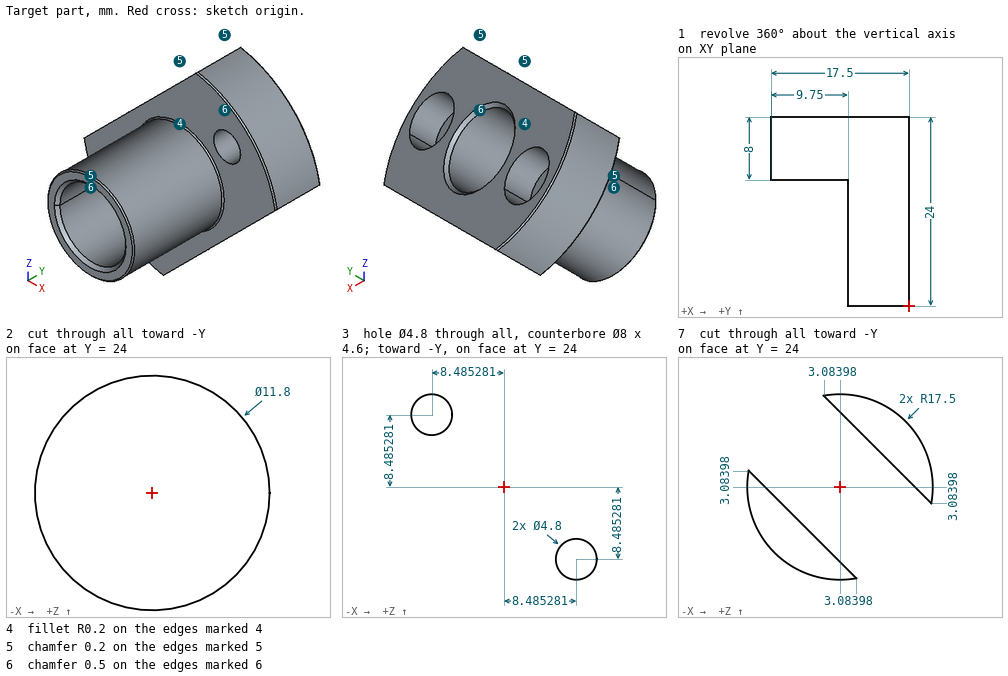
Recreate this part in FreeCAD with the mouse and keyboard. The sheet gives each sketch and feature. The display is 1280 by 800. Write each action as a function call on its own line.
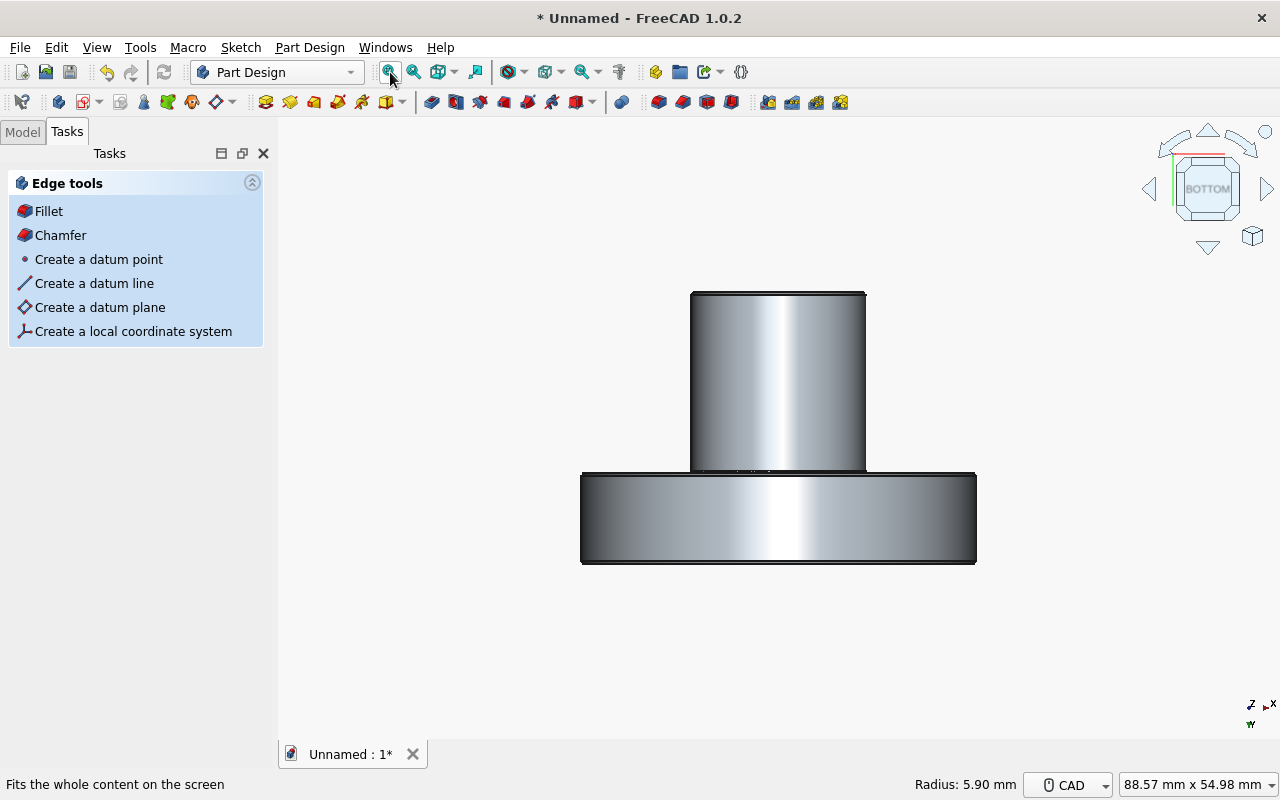
key(v)
key(f)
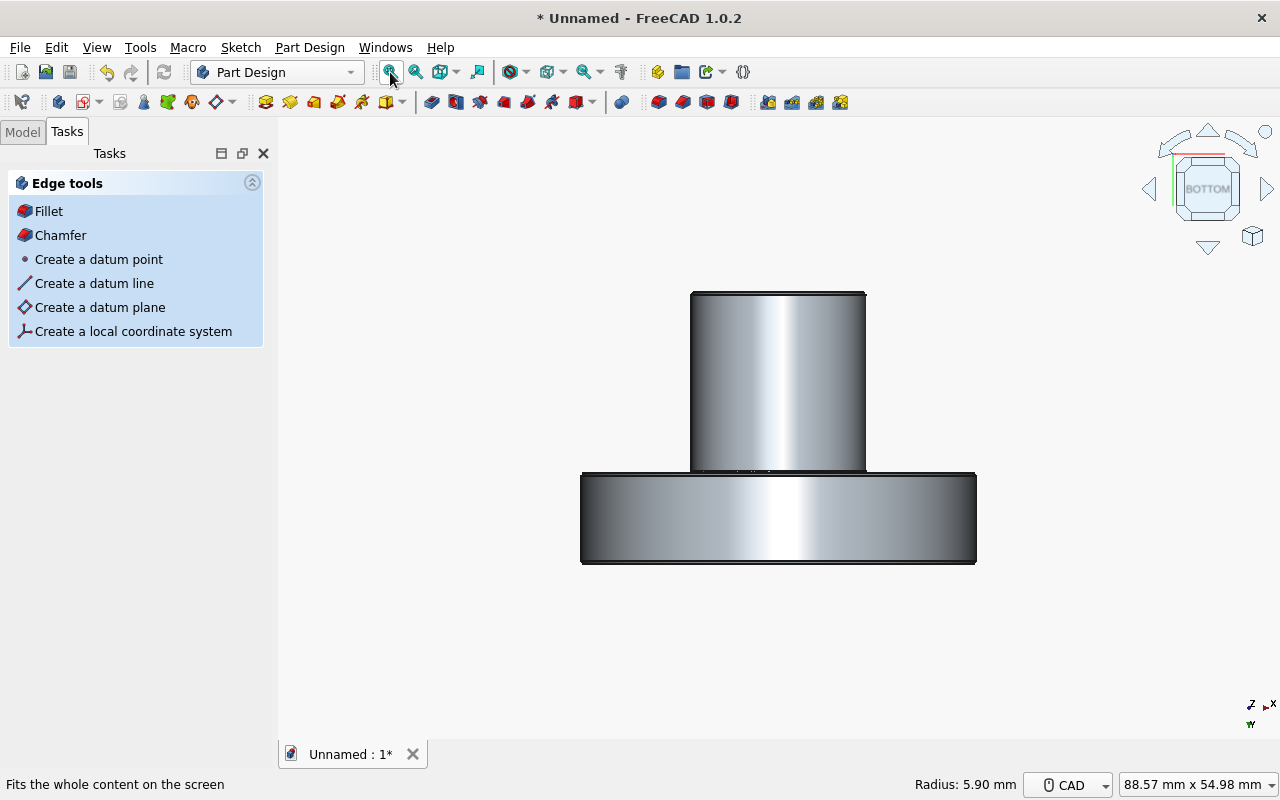
key(4)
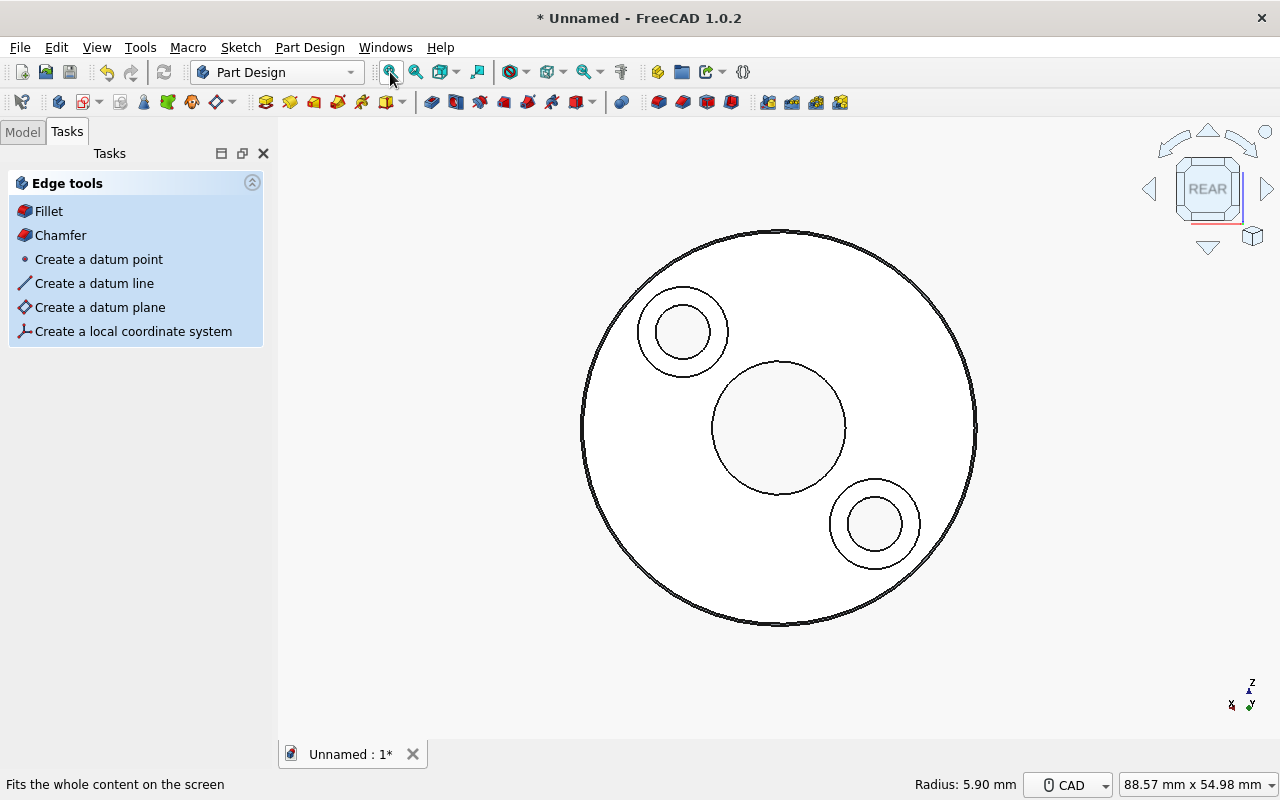
click(712, 427, ctrl)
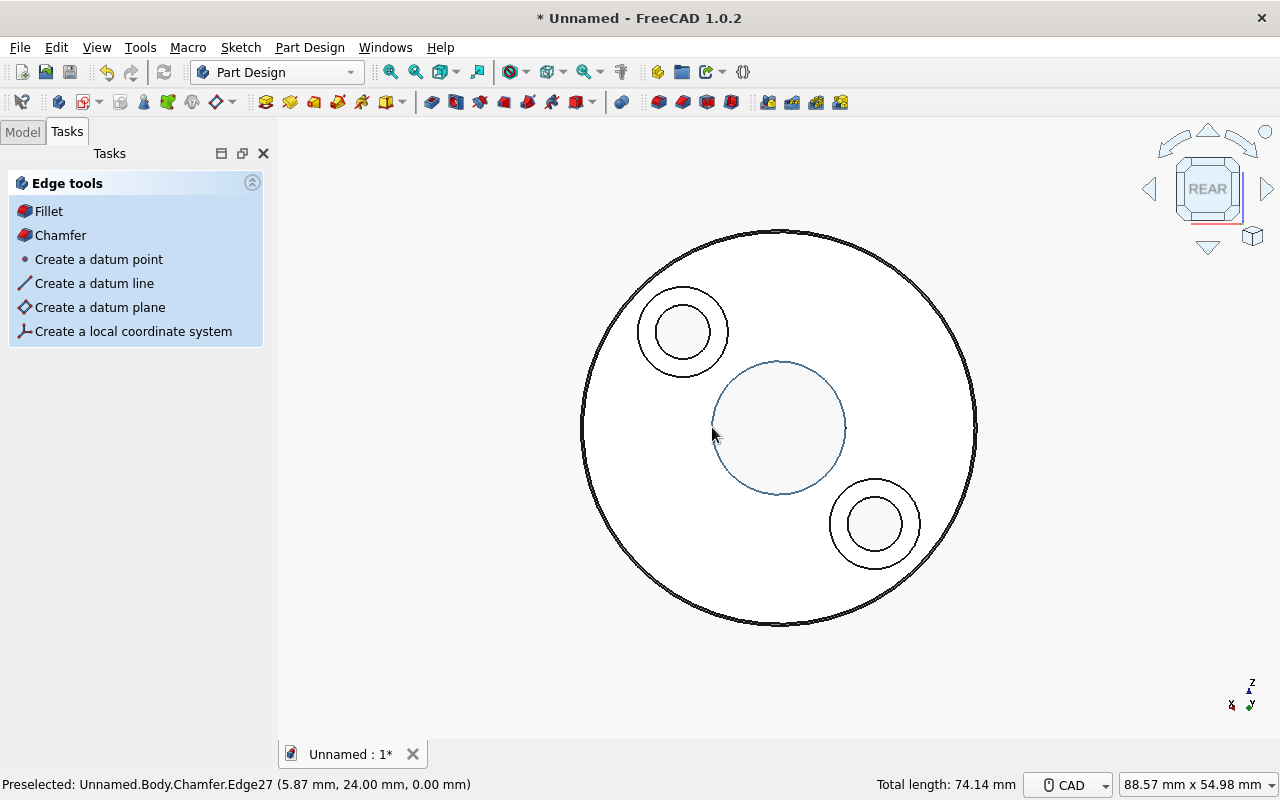
click(684, 102)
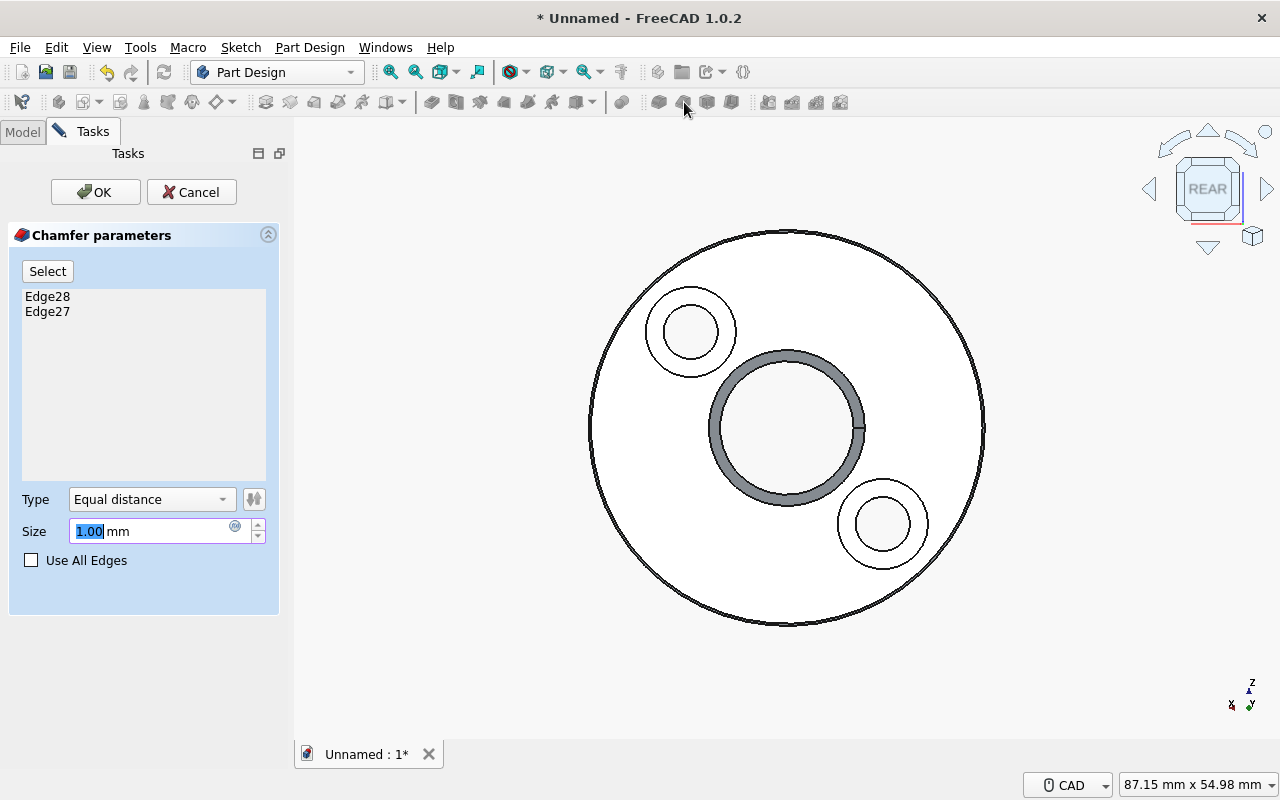
text(0.5)
key(Tab)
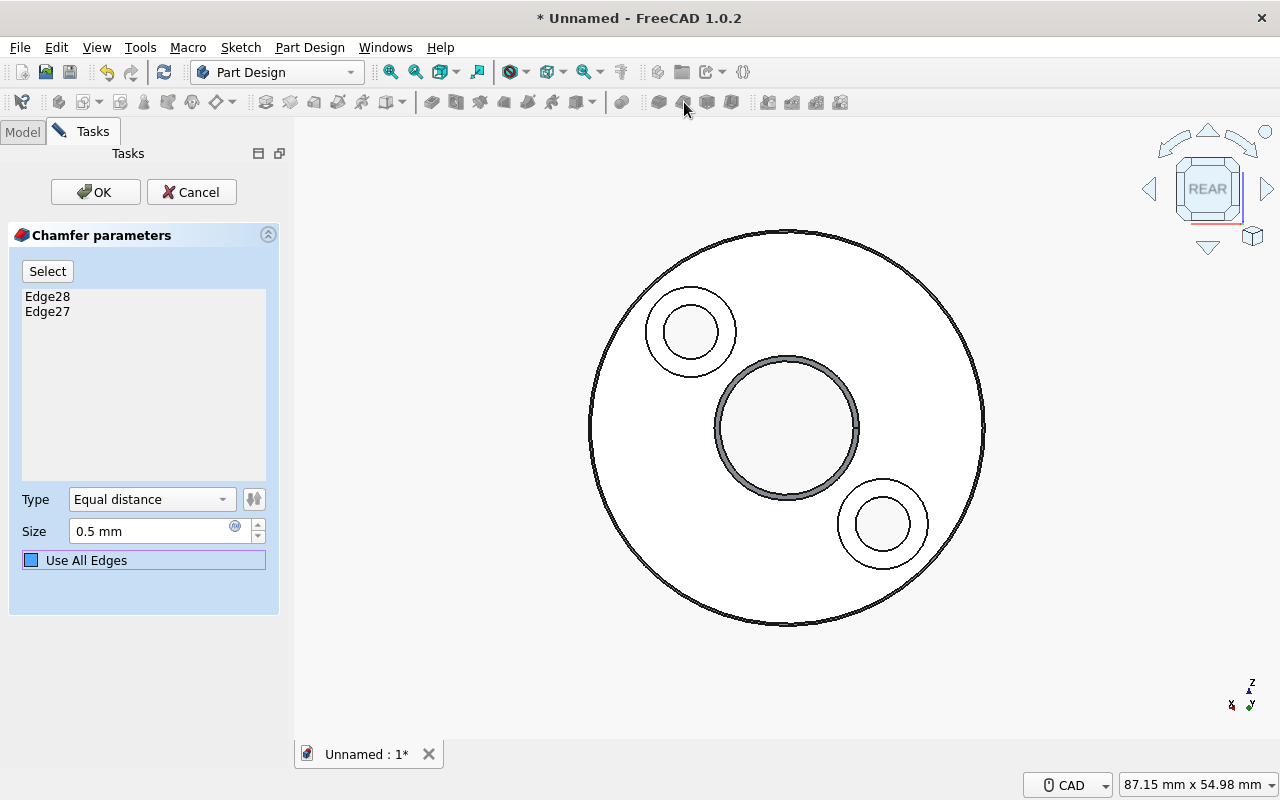
click(96, 192)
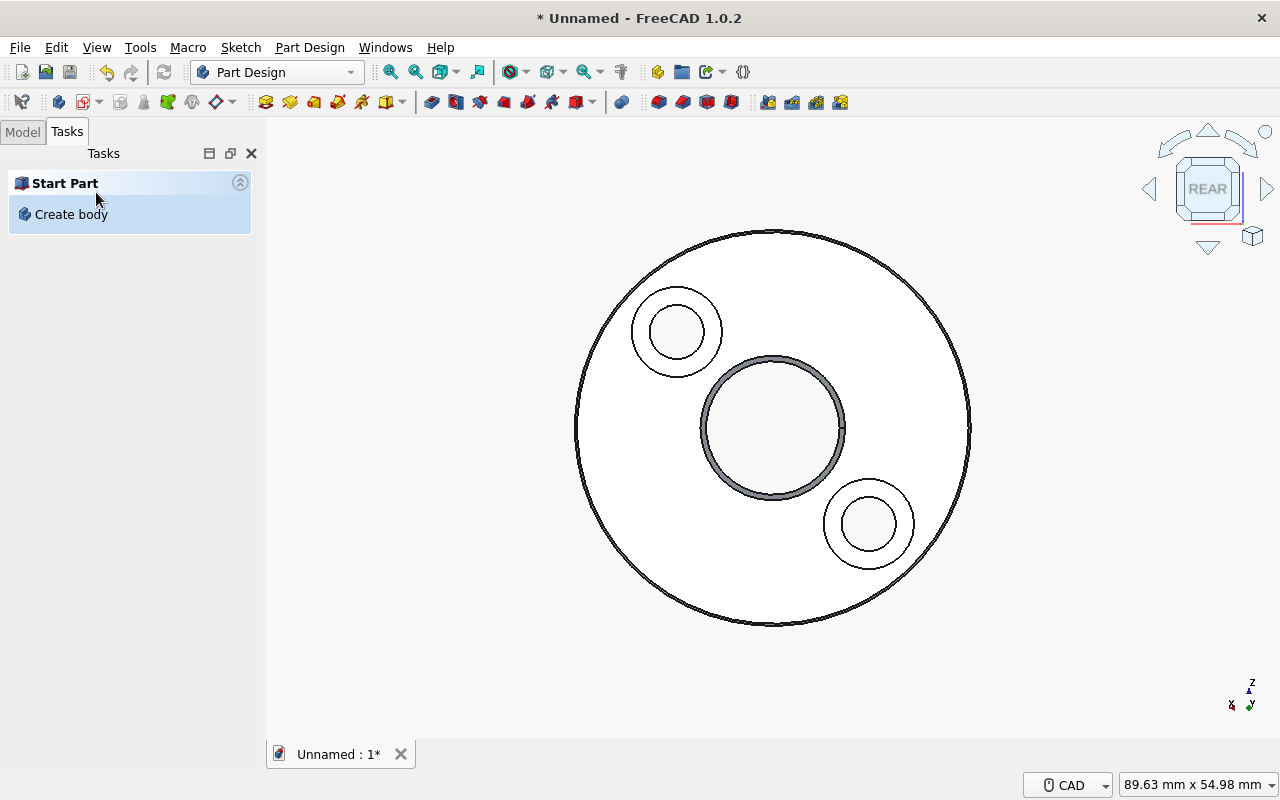
click(717, 539)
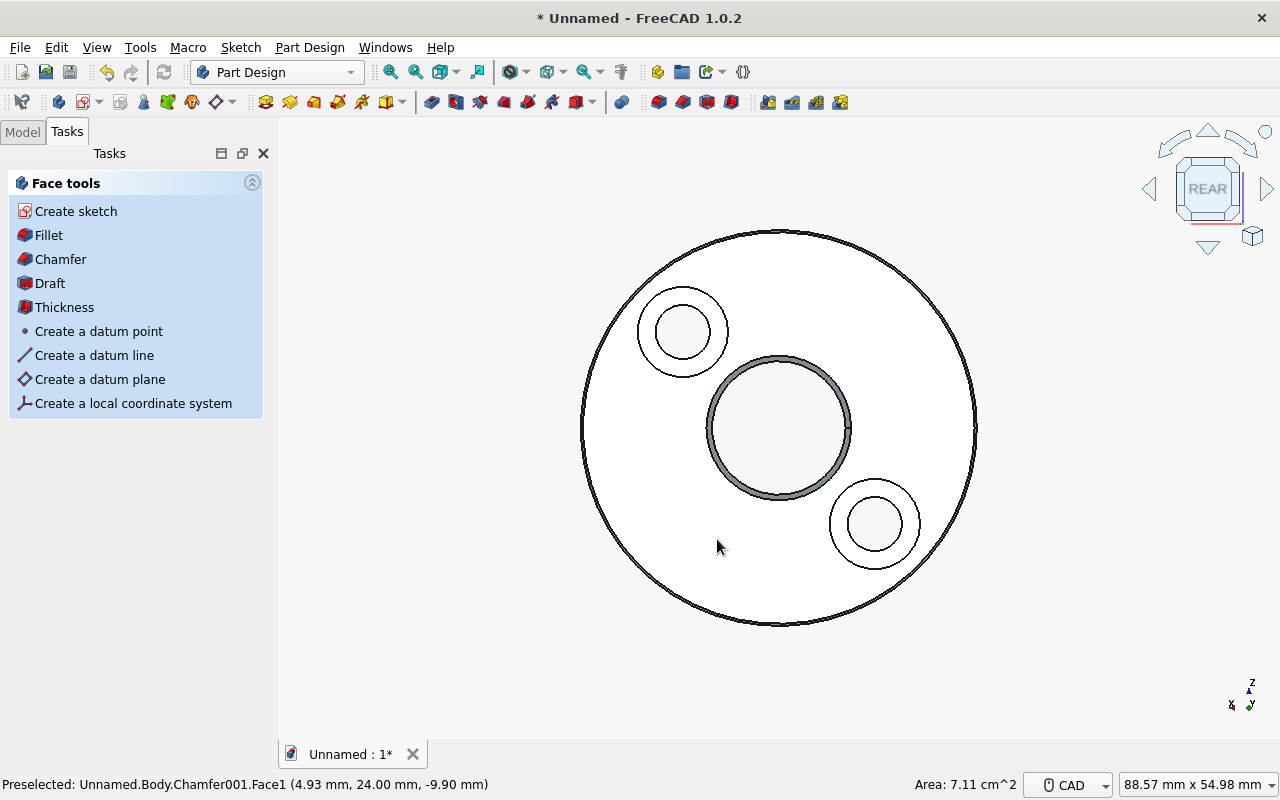
click(84, 102)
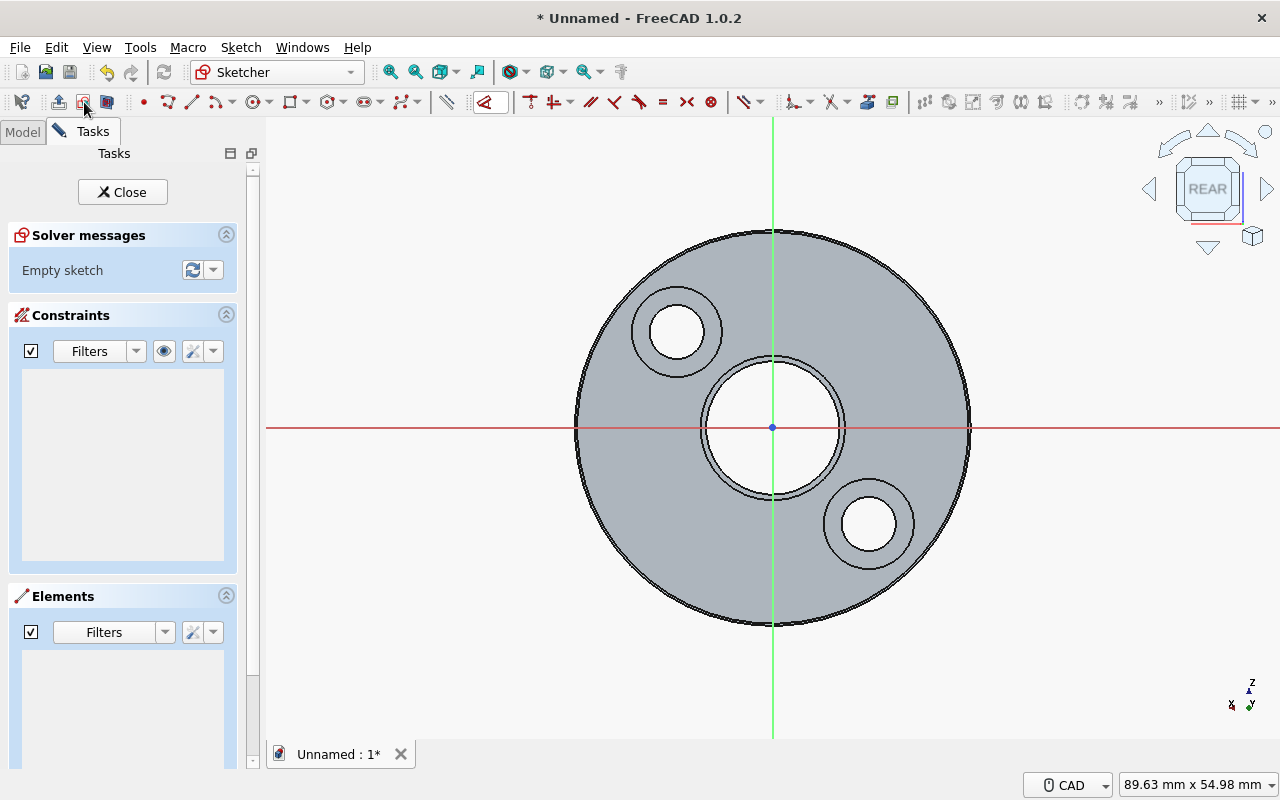
click(192, 102)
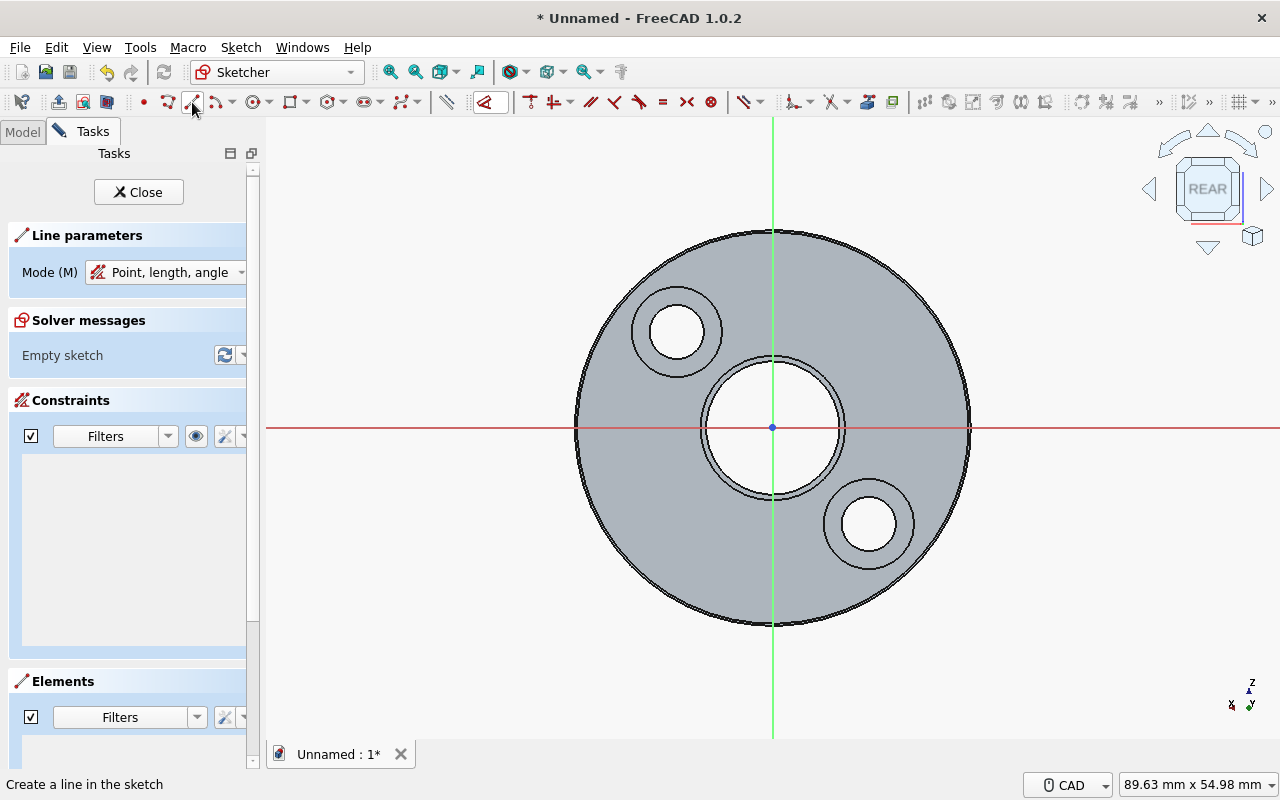
click(738, 233)
click(968, 463)